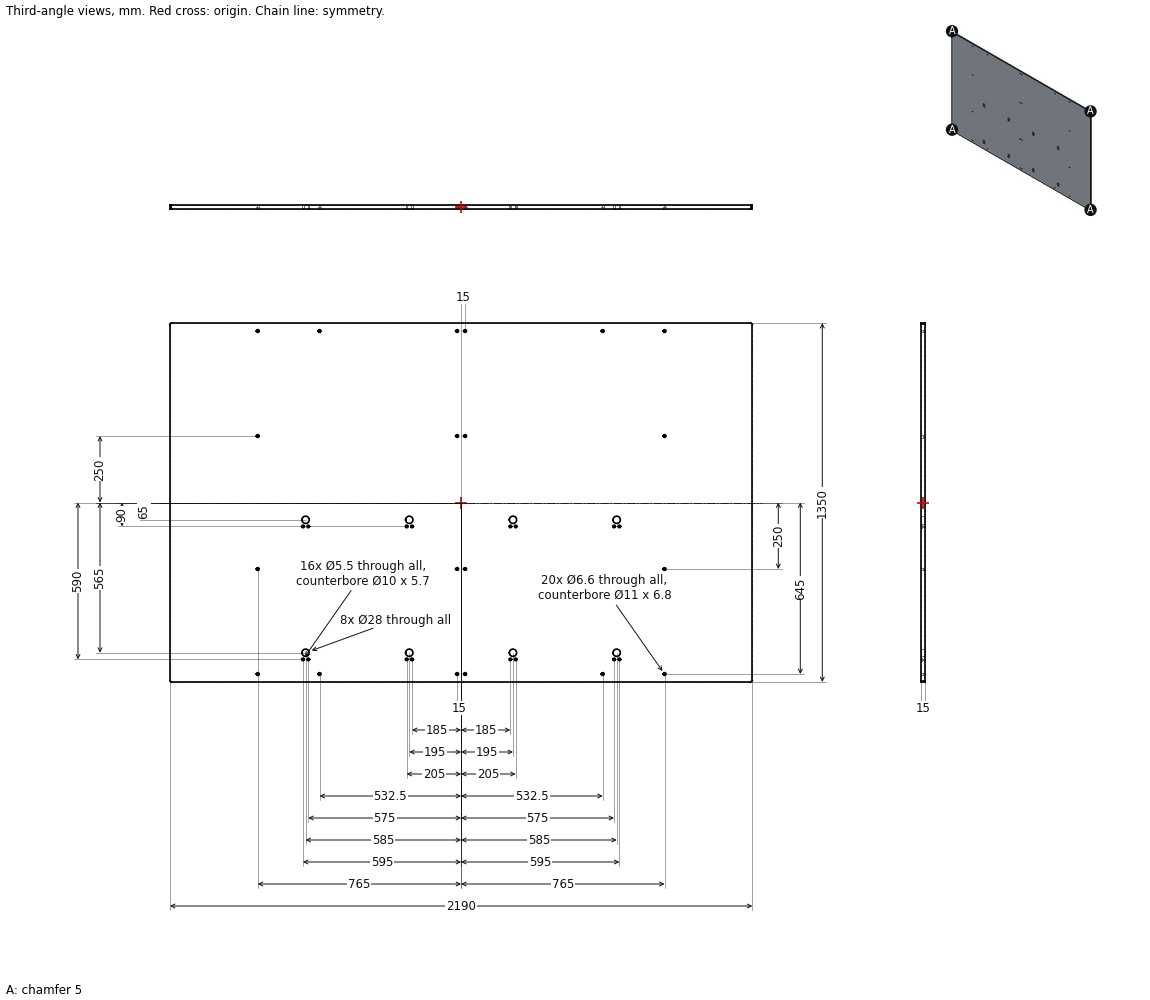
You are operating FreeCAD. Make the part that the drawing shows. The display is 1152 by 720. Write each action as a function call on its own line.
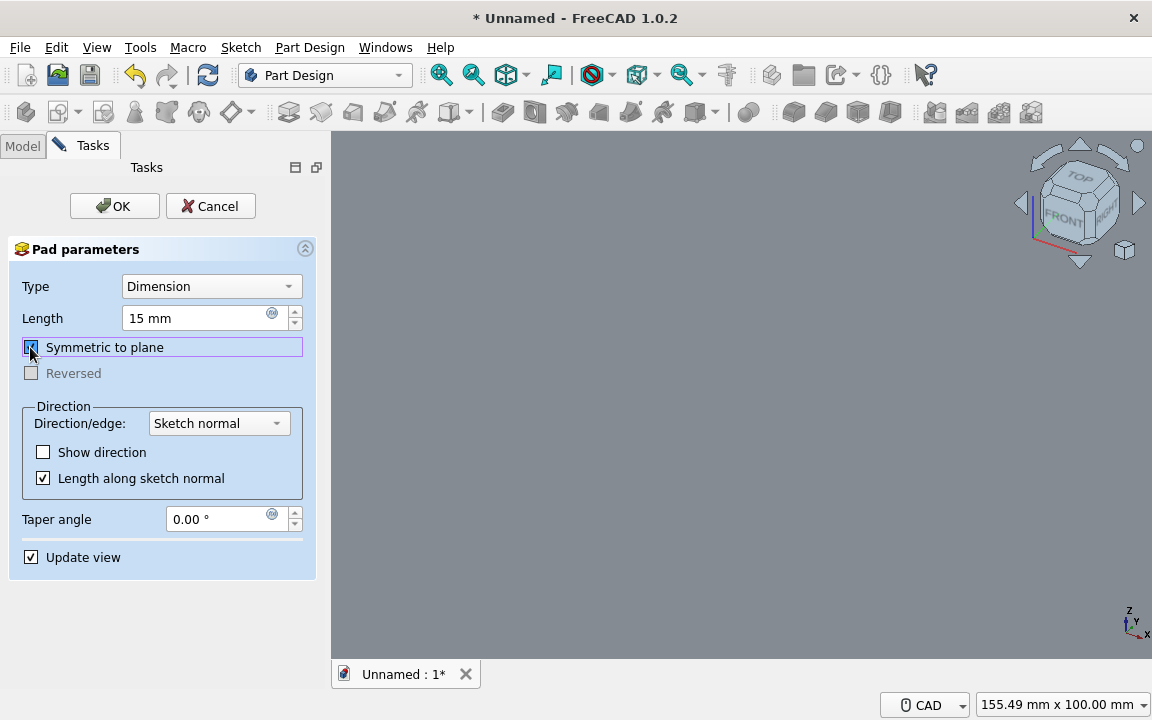
click(115, 206)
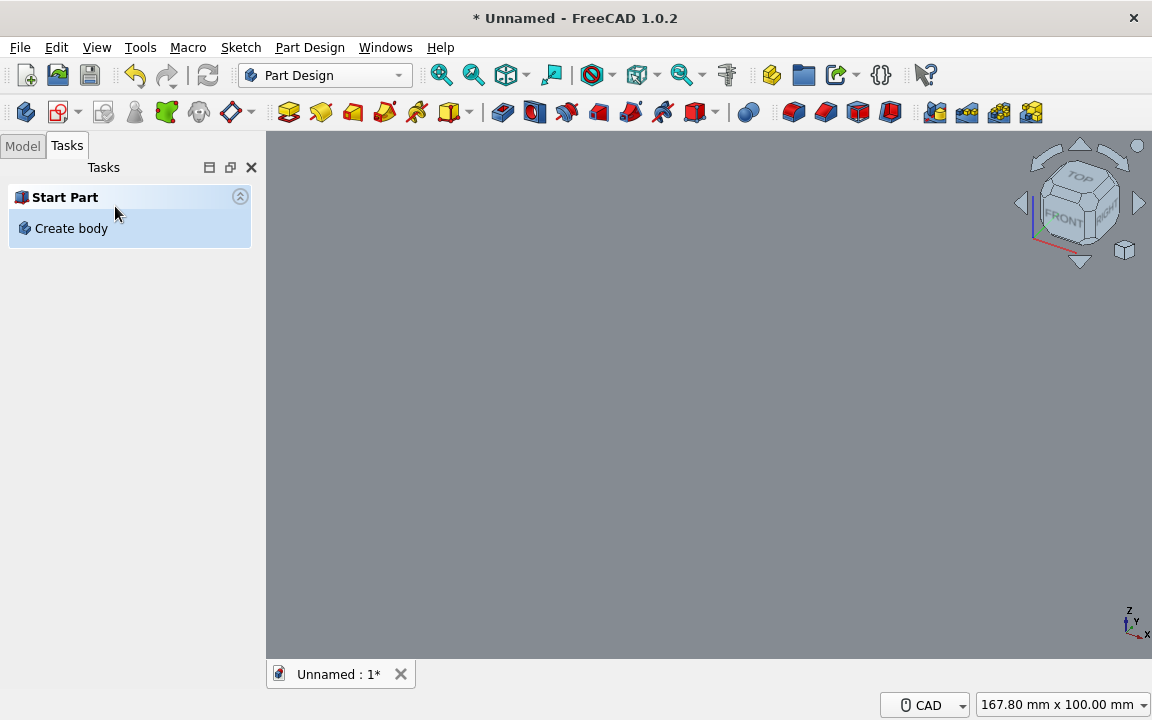
click(442, 76)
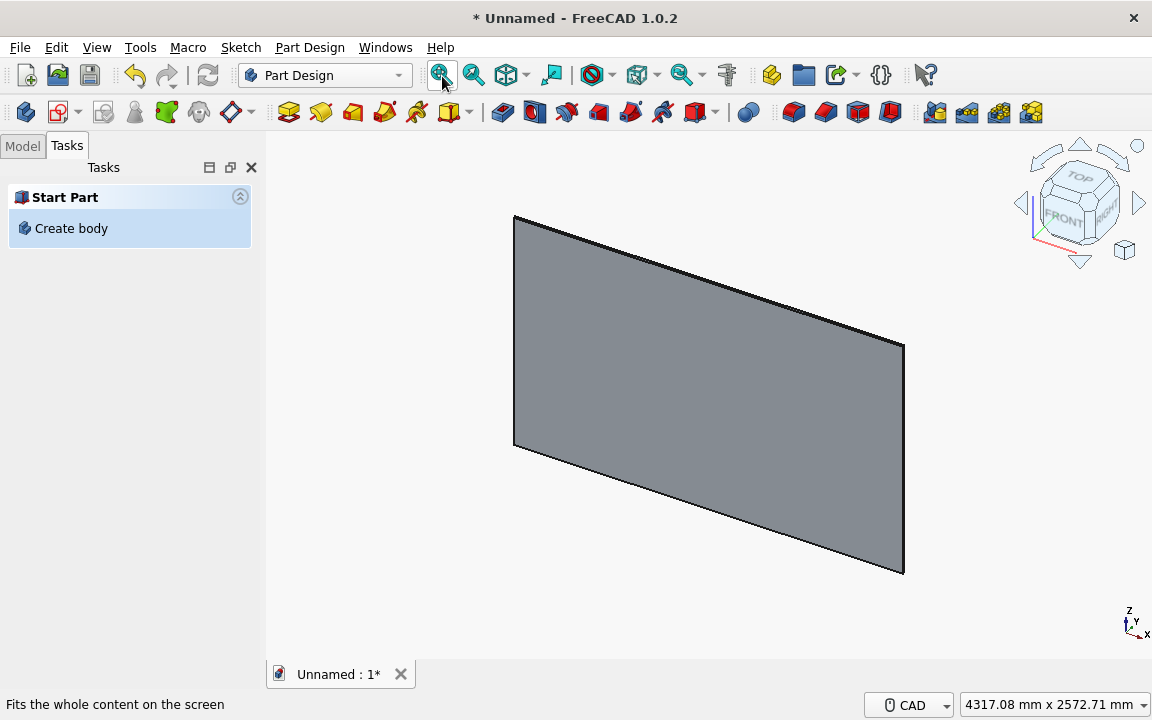
scroll(904, 345, up, 13)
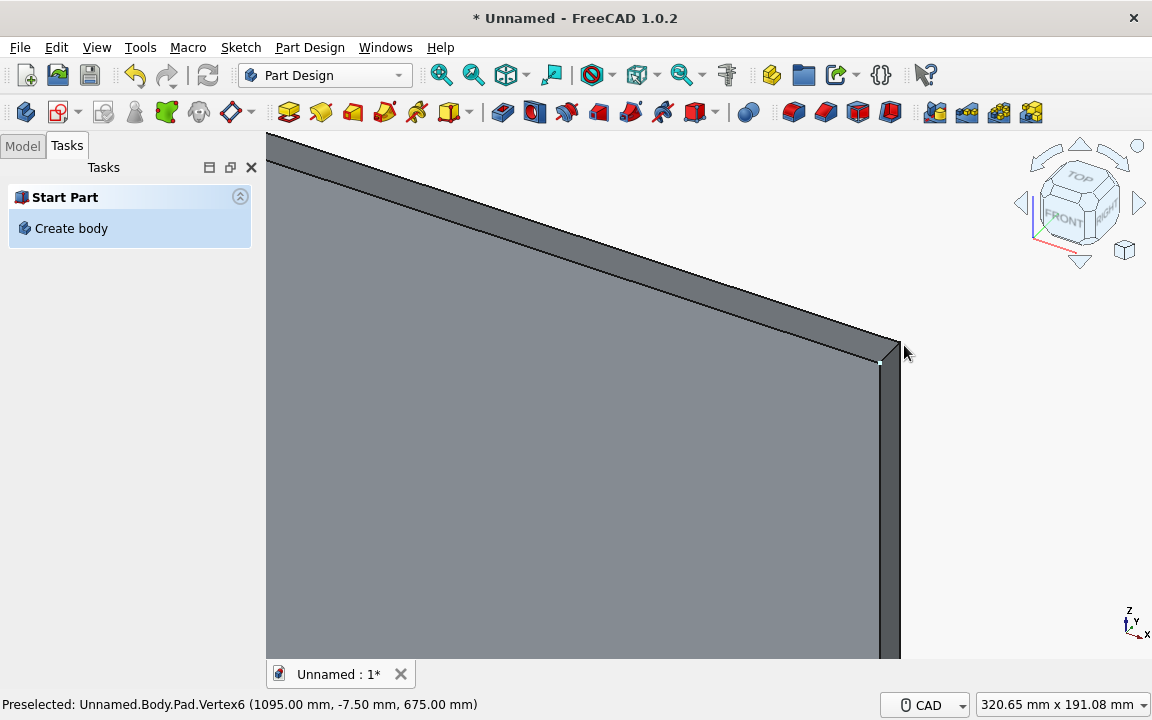
click(890, 352)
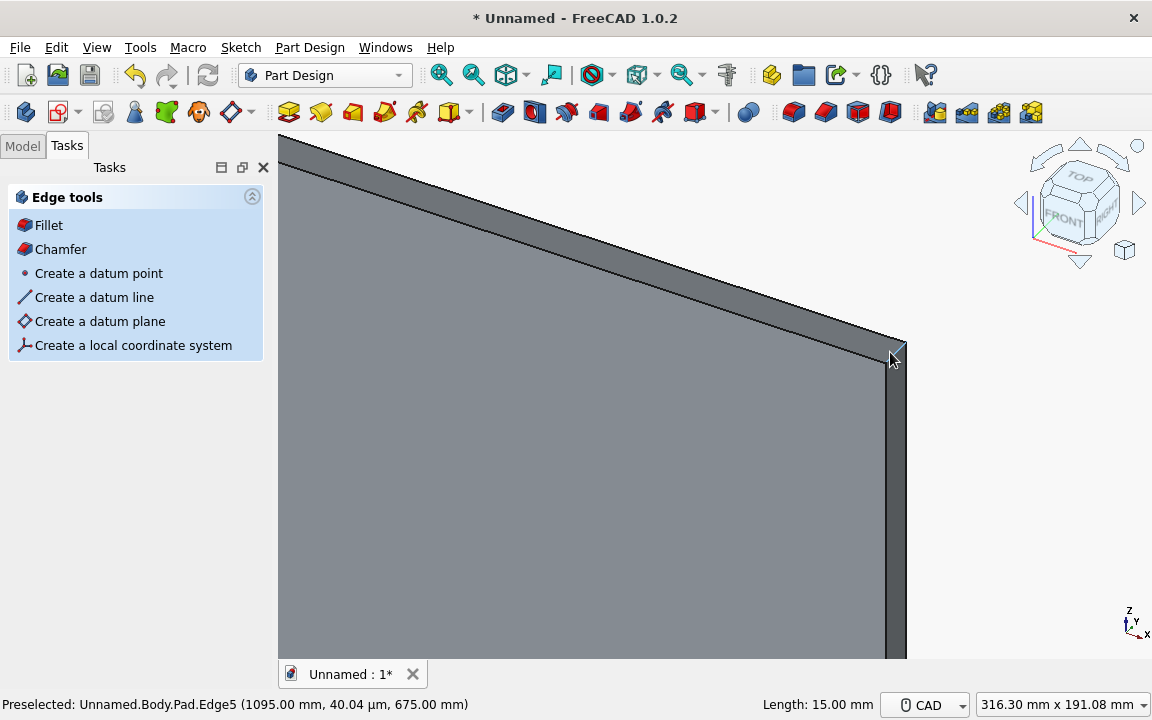
key(v)
key(f)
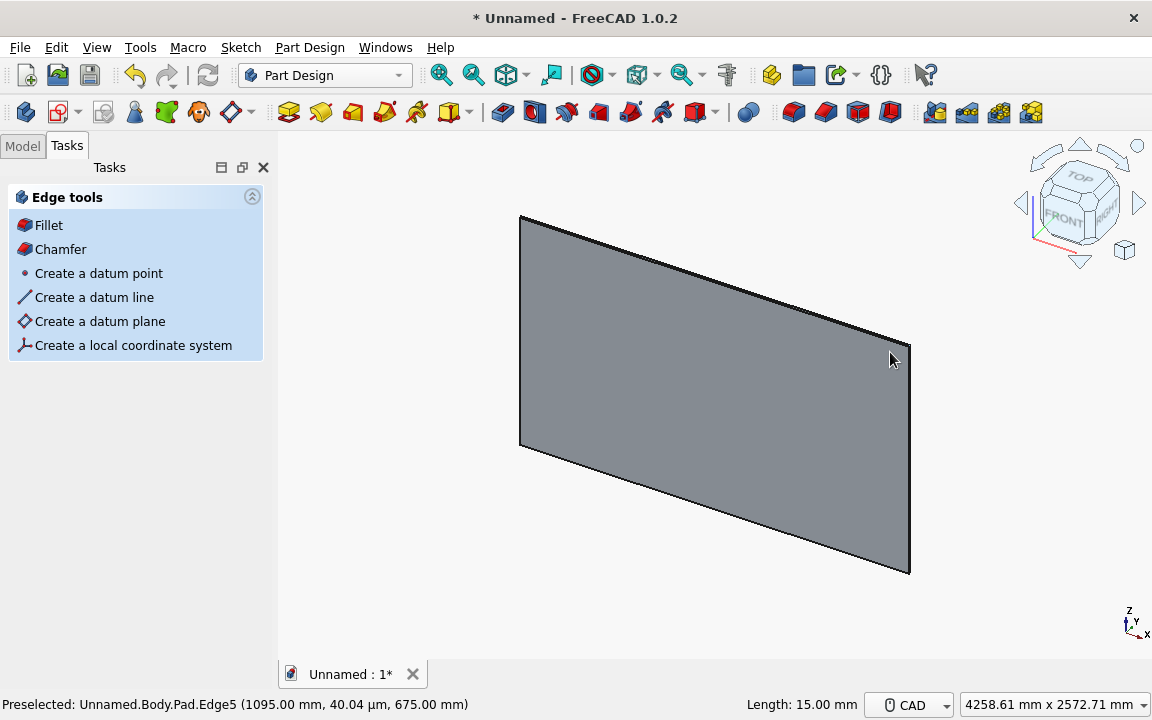
key(0)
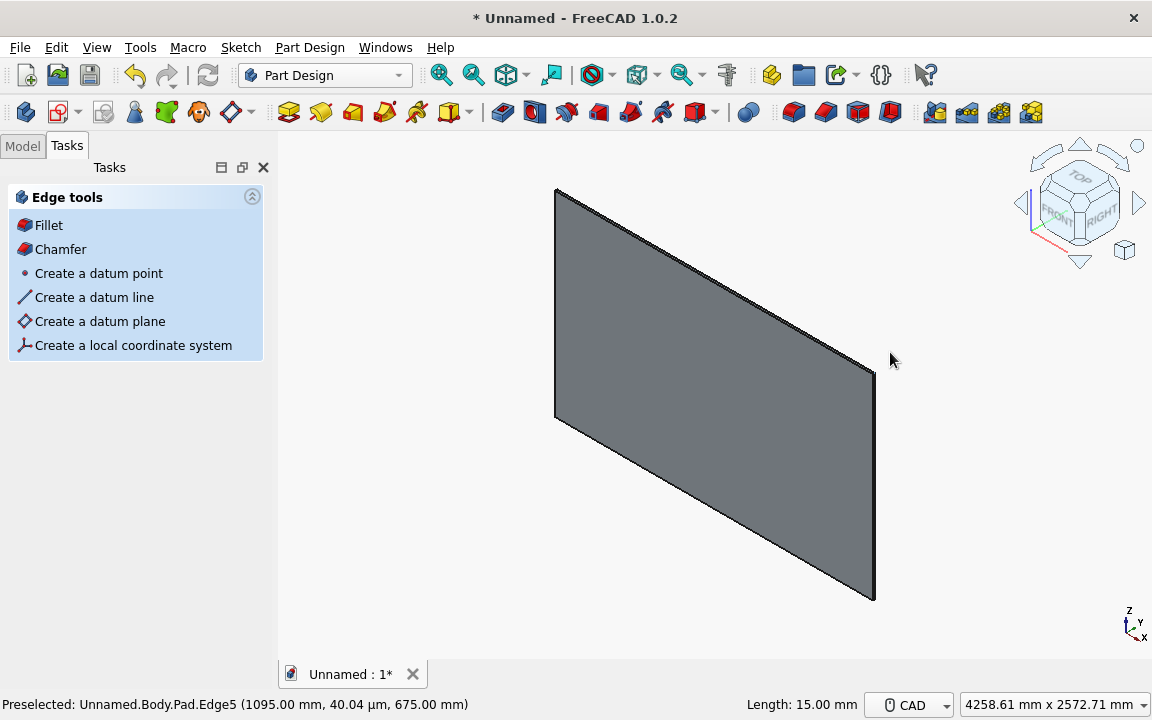
scroll(556, 189, up, 13)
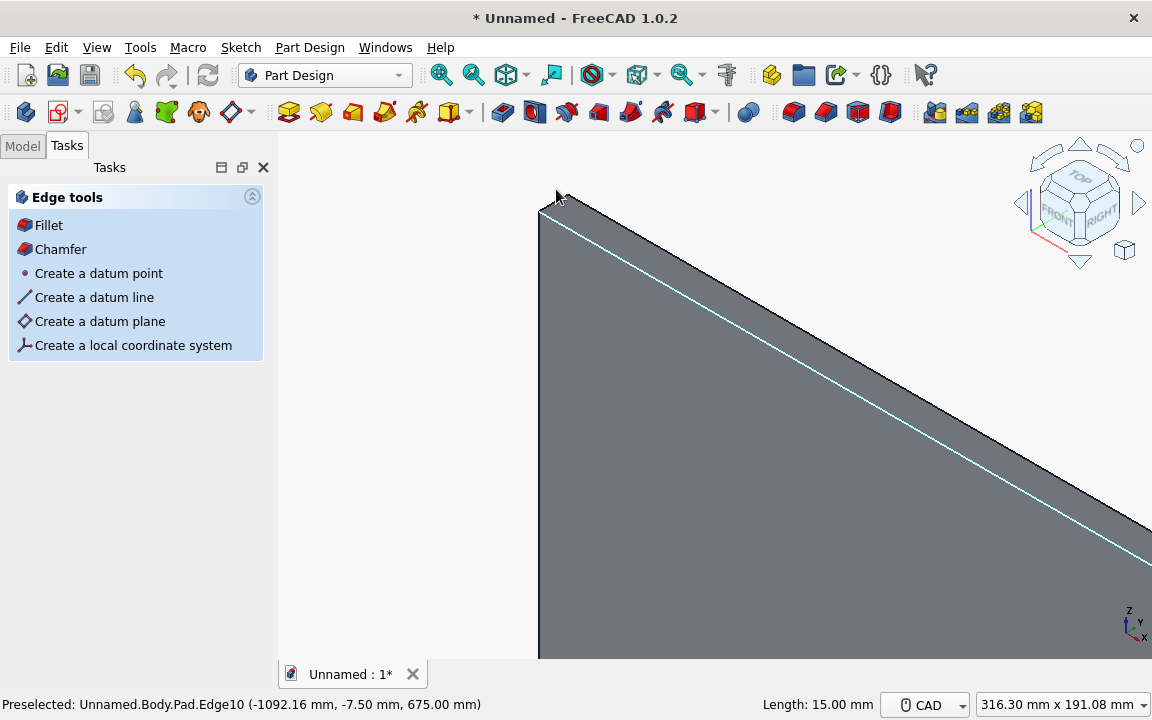
key(v)
key(f)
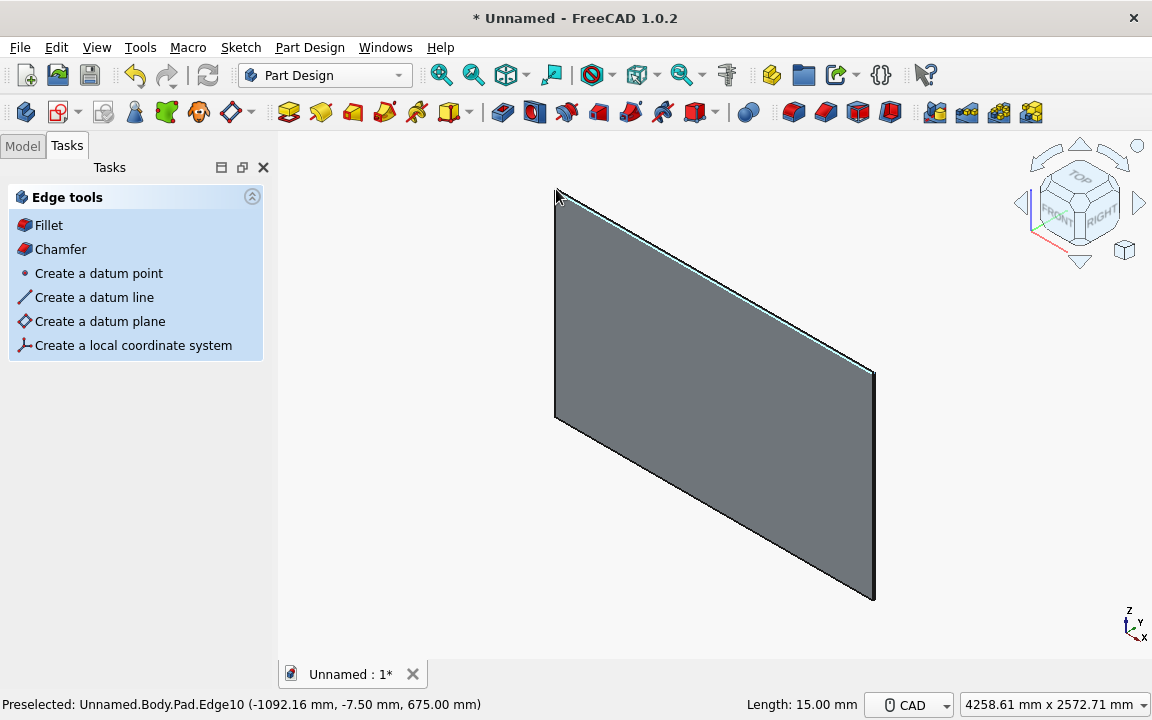
key(2)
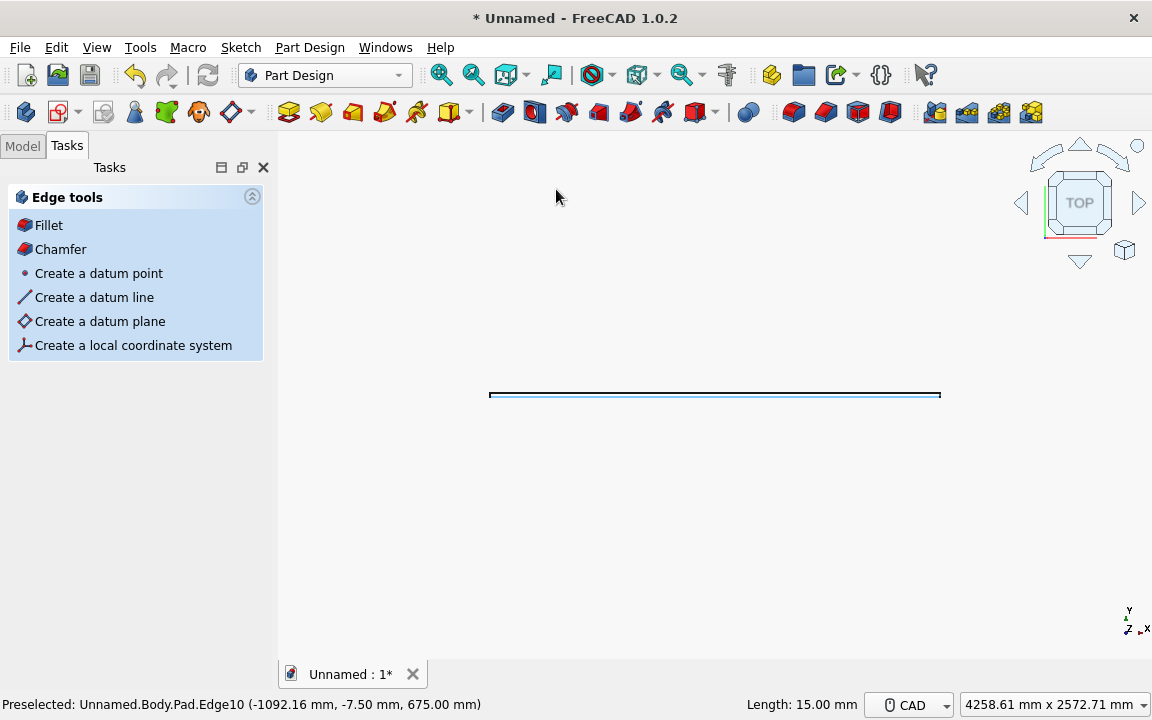
scroll(490, 394, up, 13)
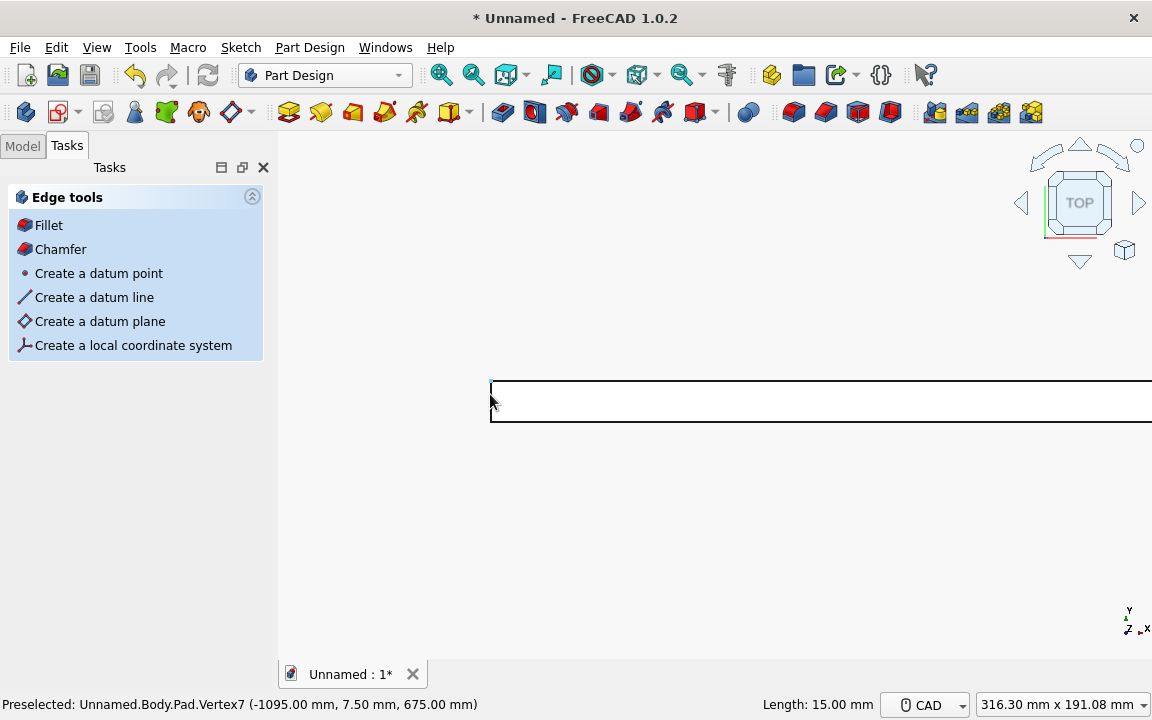
click(491, 400, ctrl)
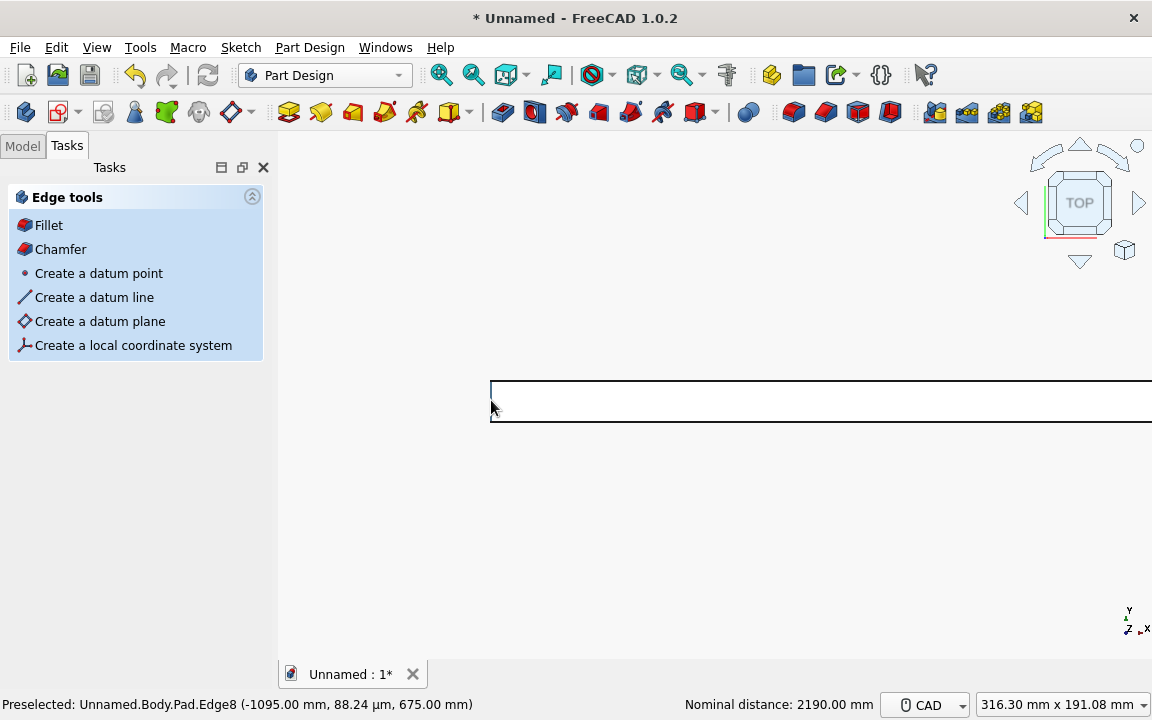
key(v)
key(f)